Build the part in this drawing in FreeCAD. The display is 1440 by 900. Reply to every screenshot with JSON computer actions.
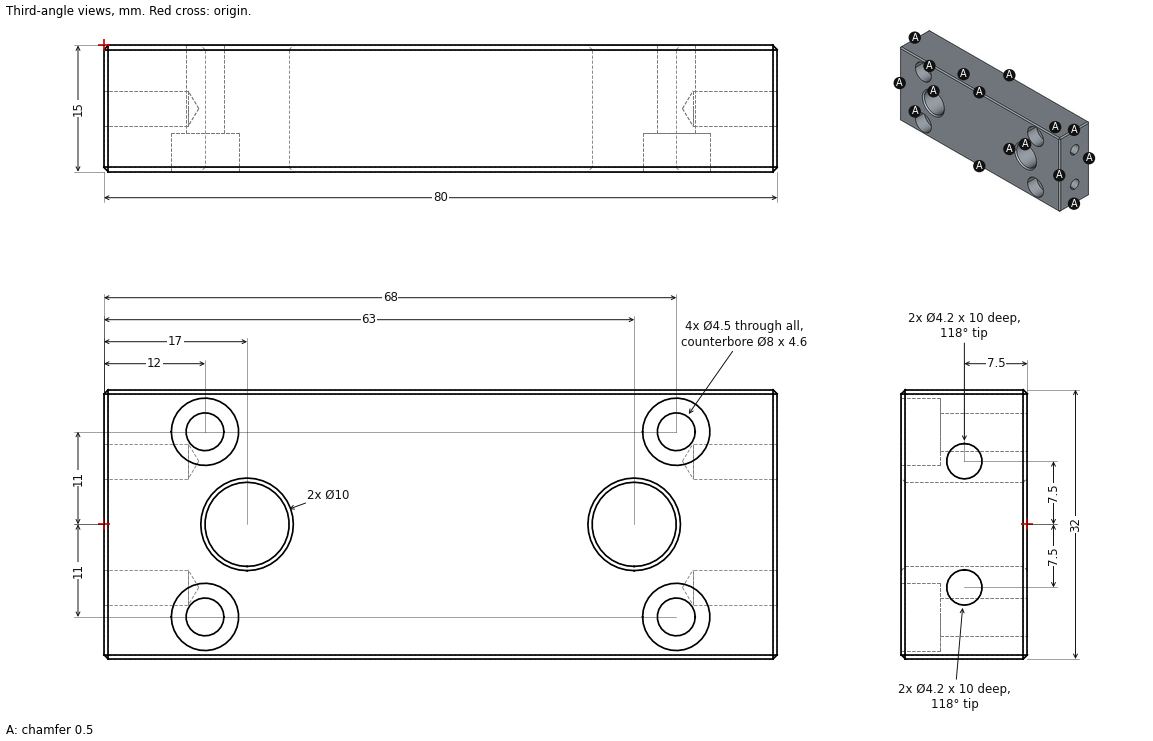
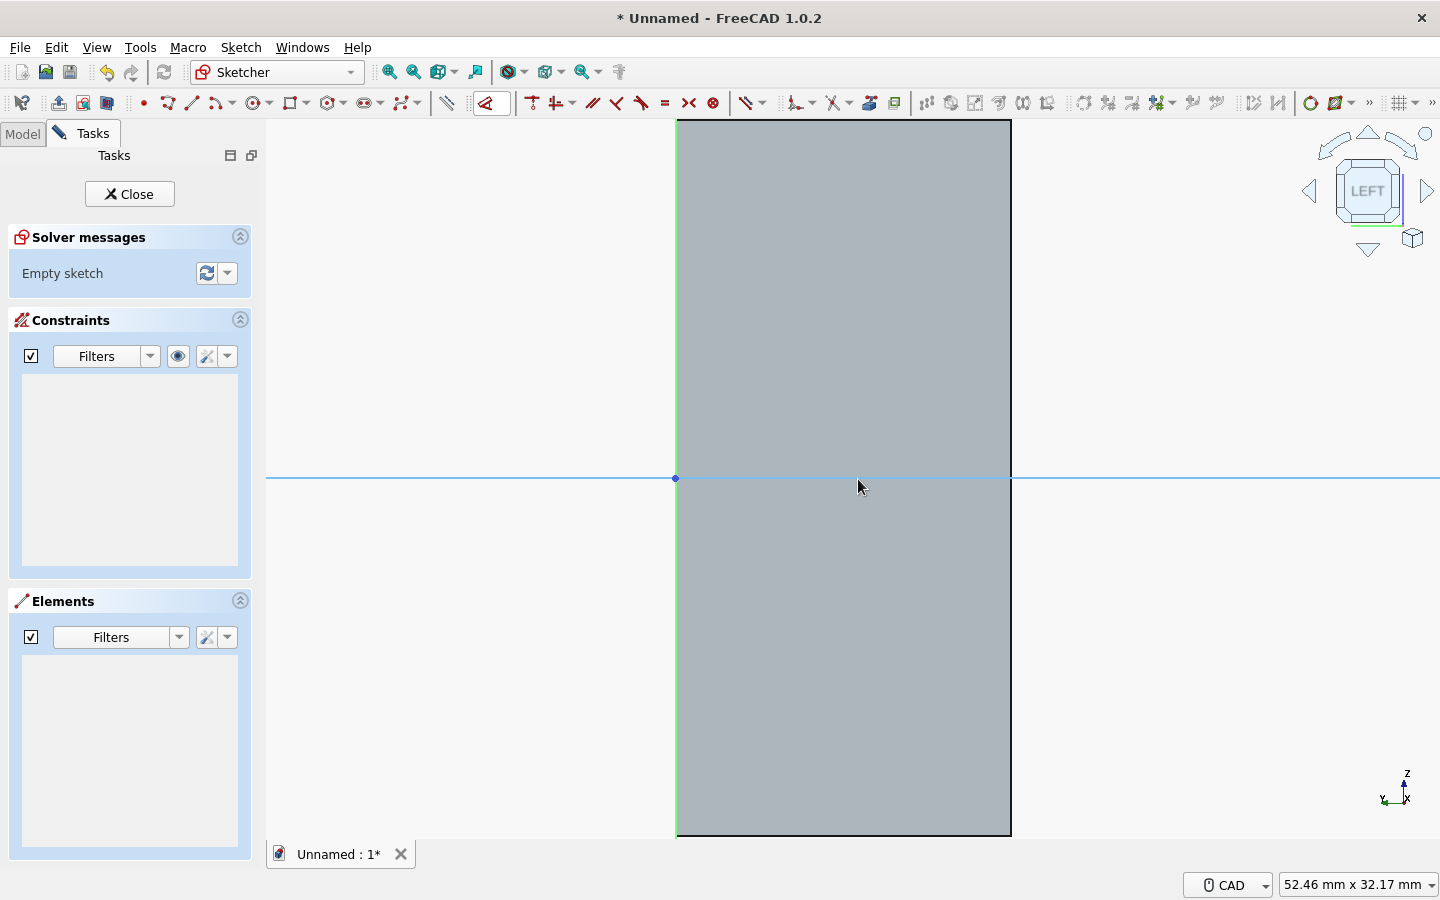
{"action": "left_click", "coordinate": [254, 104]}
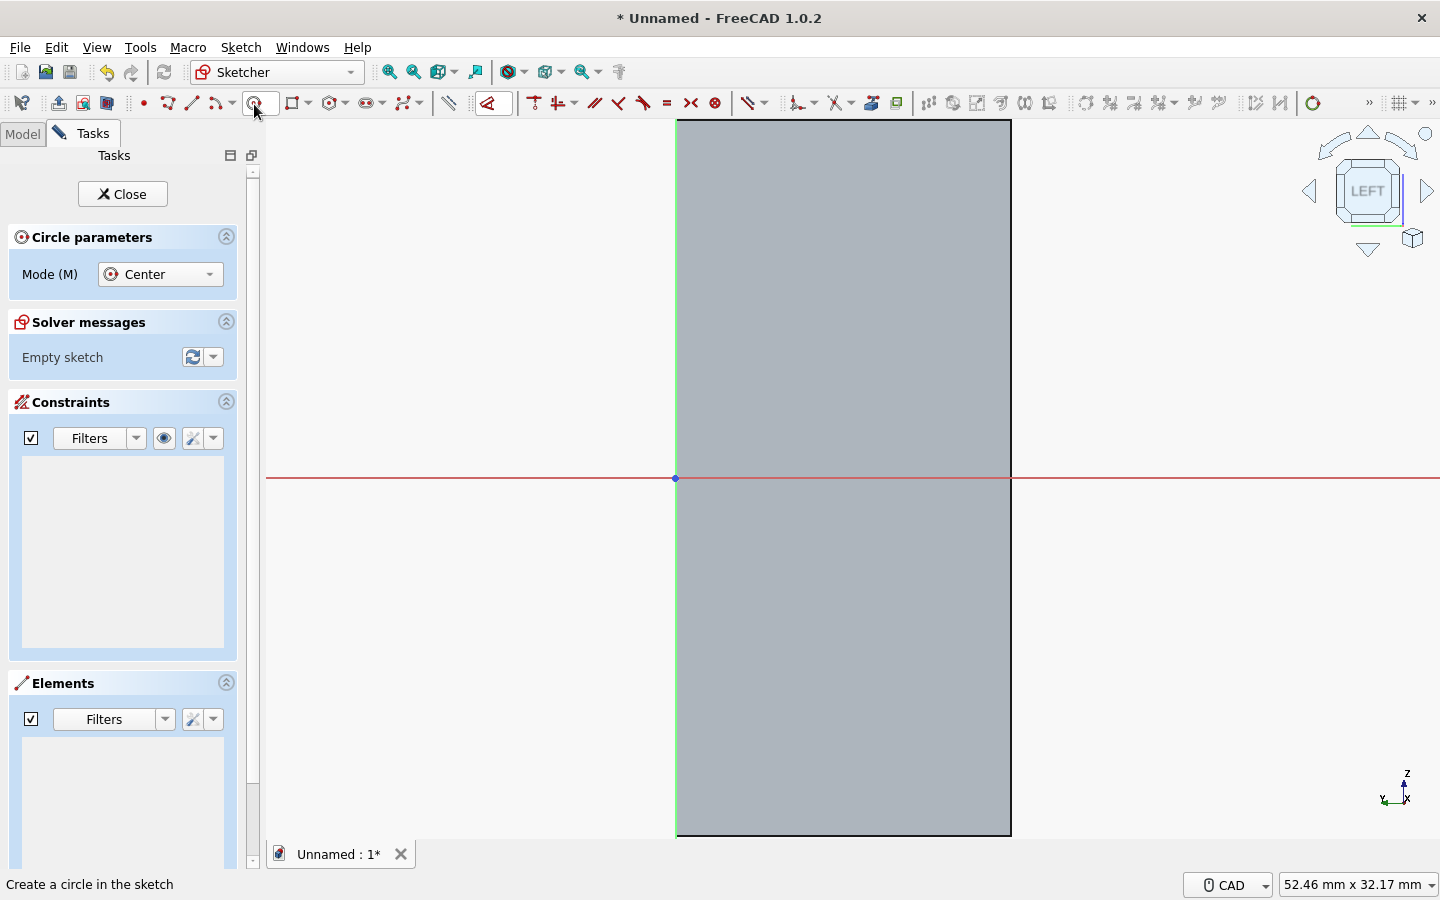
{"action": "left_click", "coordinate": [844, 646]}
{"action": "left_click", "coordinate": [877, 613]}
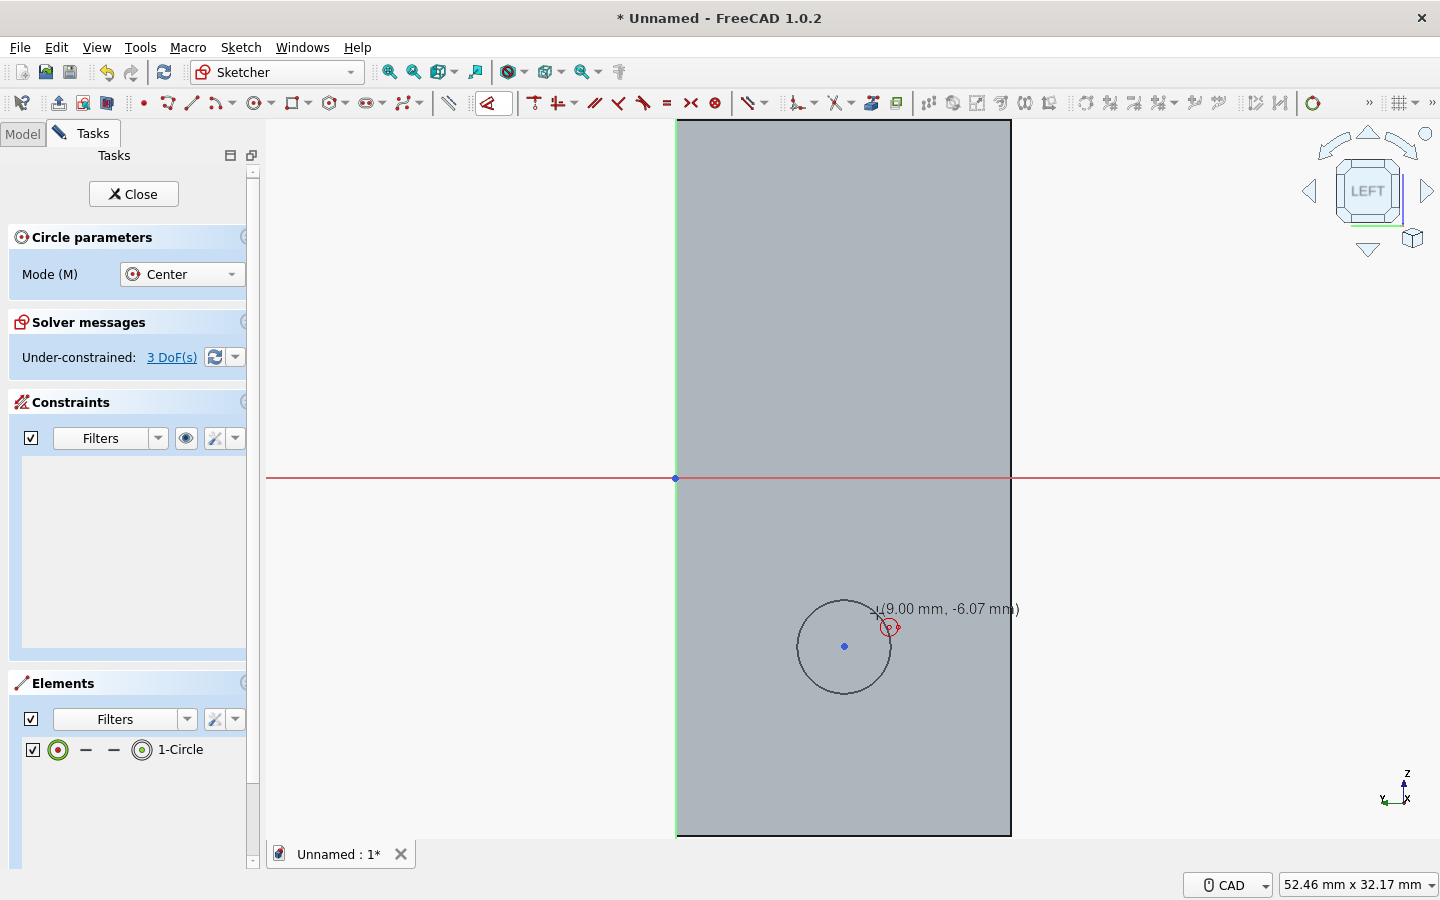
{"action": "left_click", "coordinate": [844, 310]}
{"action": "left_click", "coordinate": [877, 277]}
{"action": "key", "text": "Escape"}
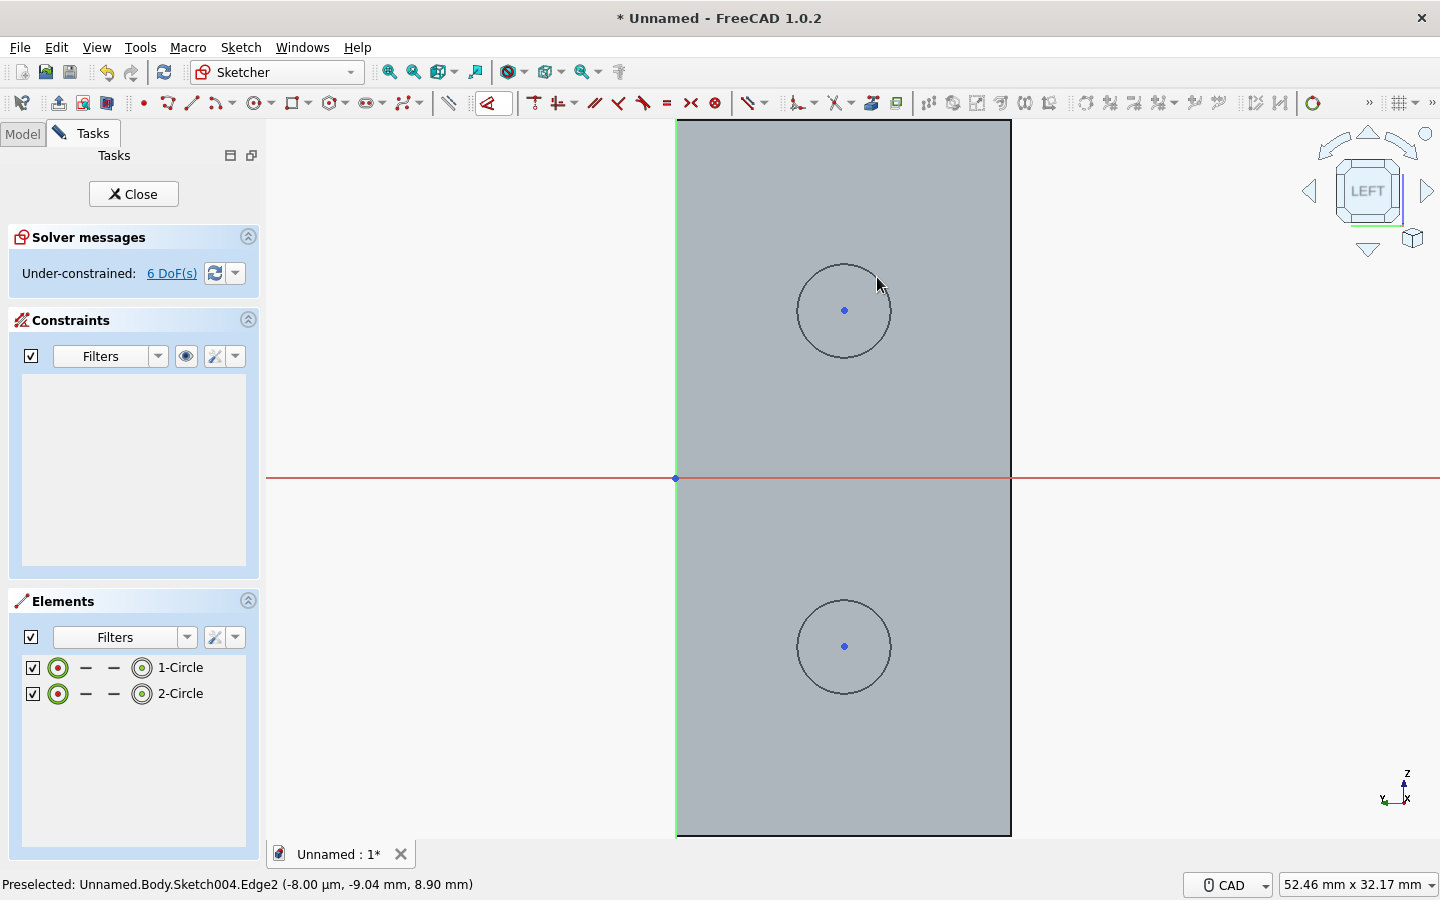
{"action": "left_click", "coordinate": [877, 614]}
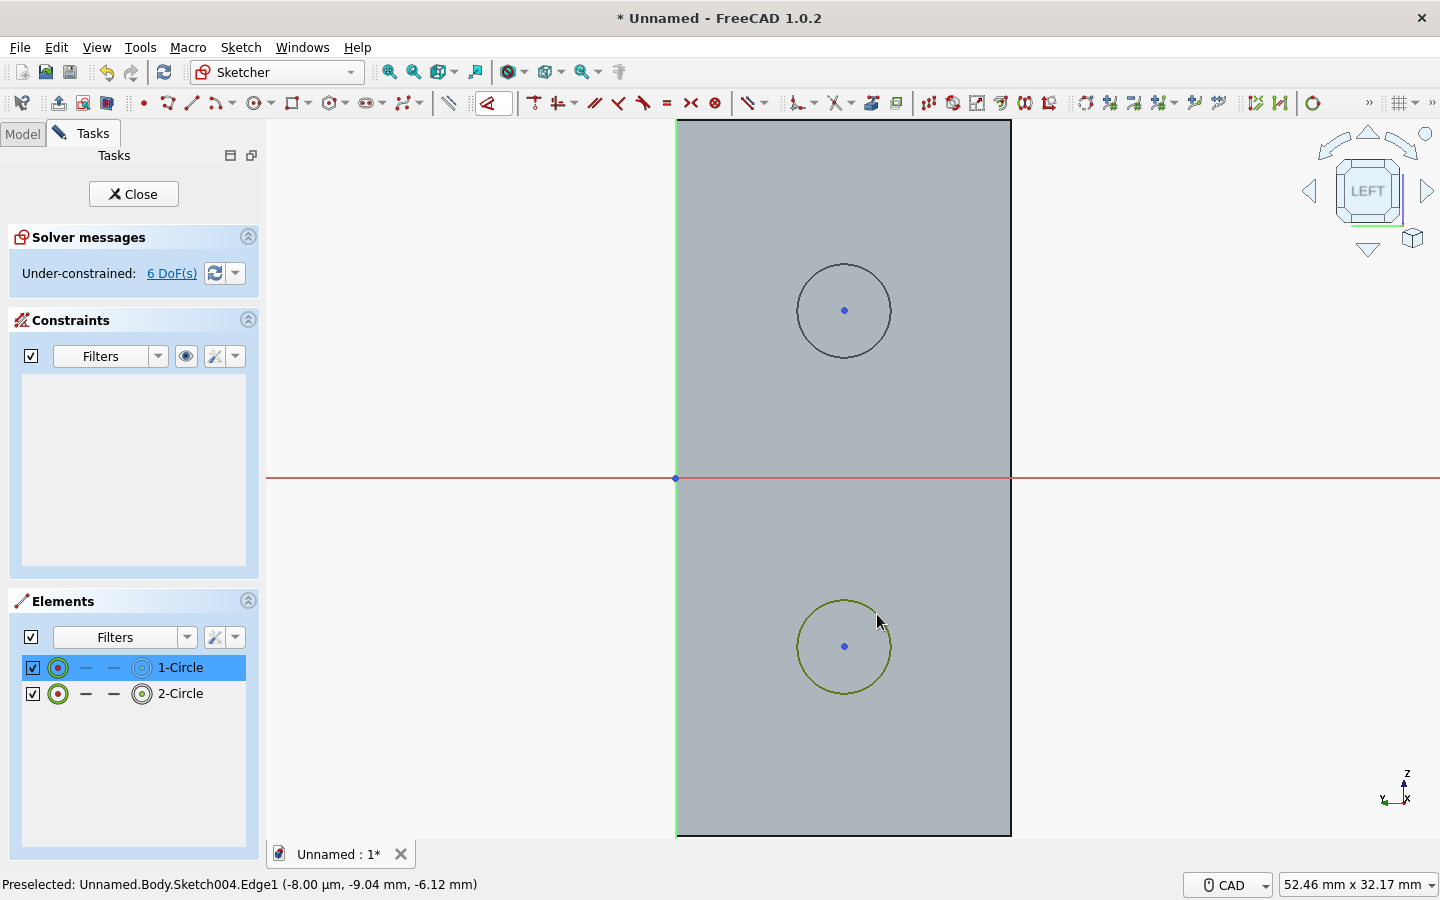
{"action": "left_click", "coordinate": [877, 278]}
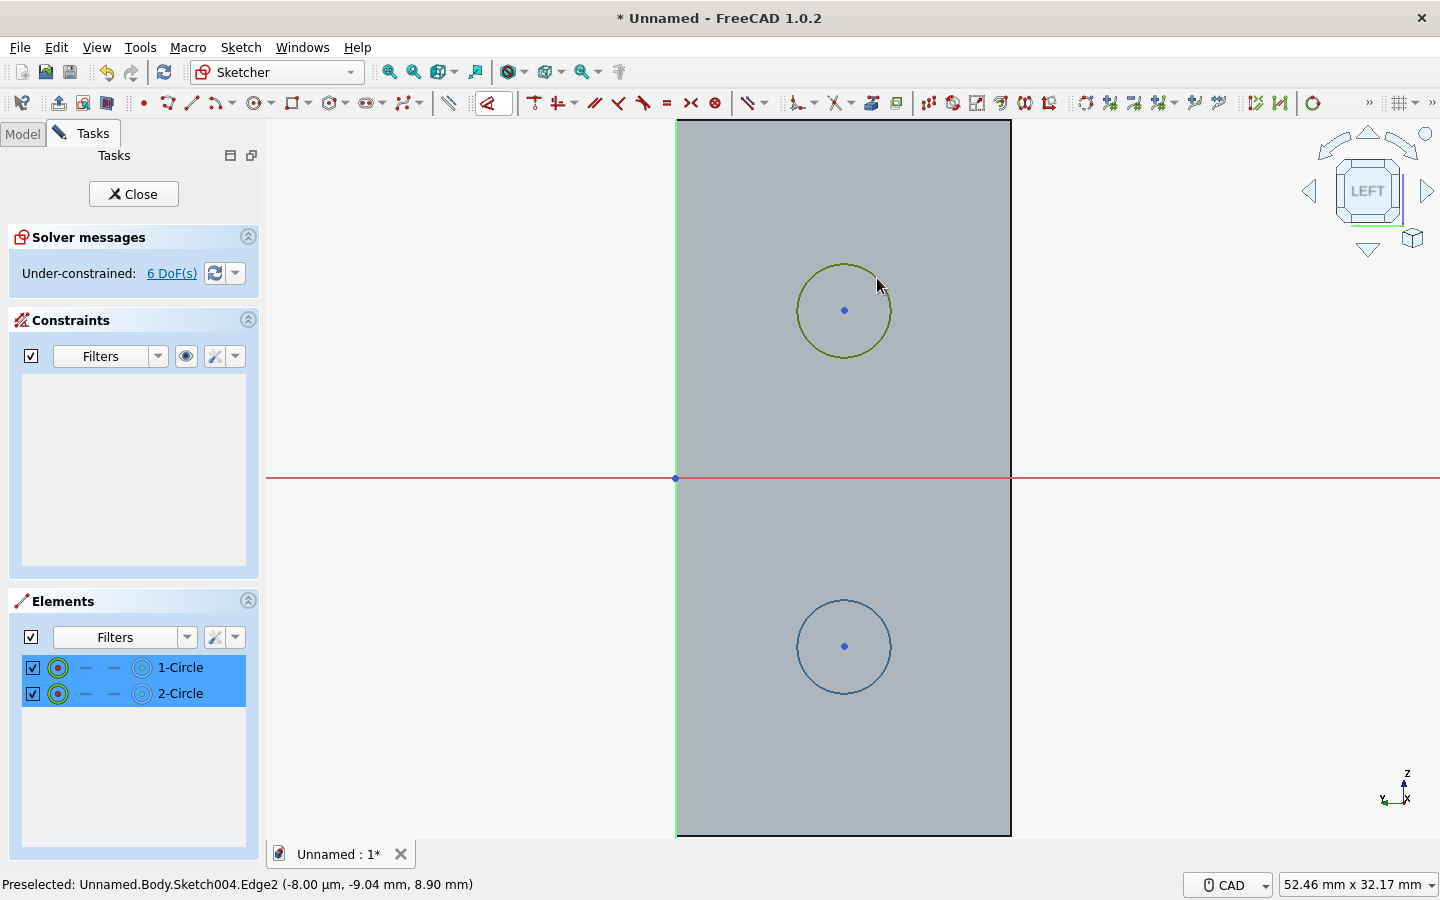
{"action": "left_click", "coordinate": [668, 104]}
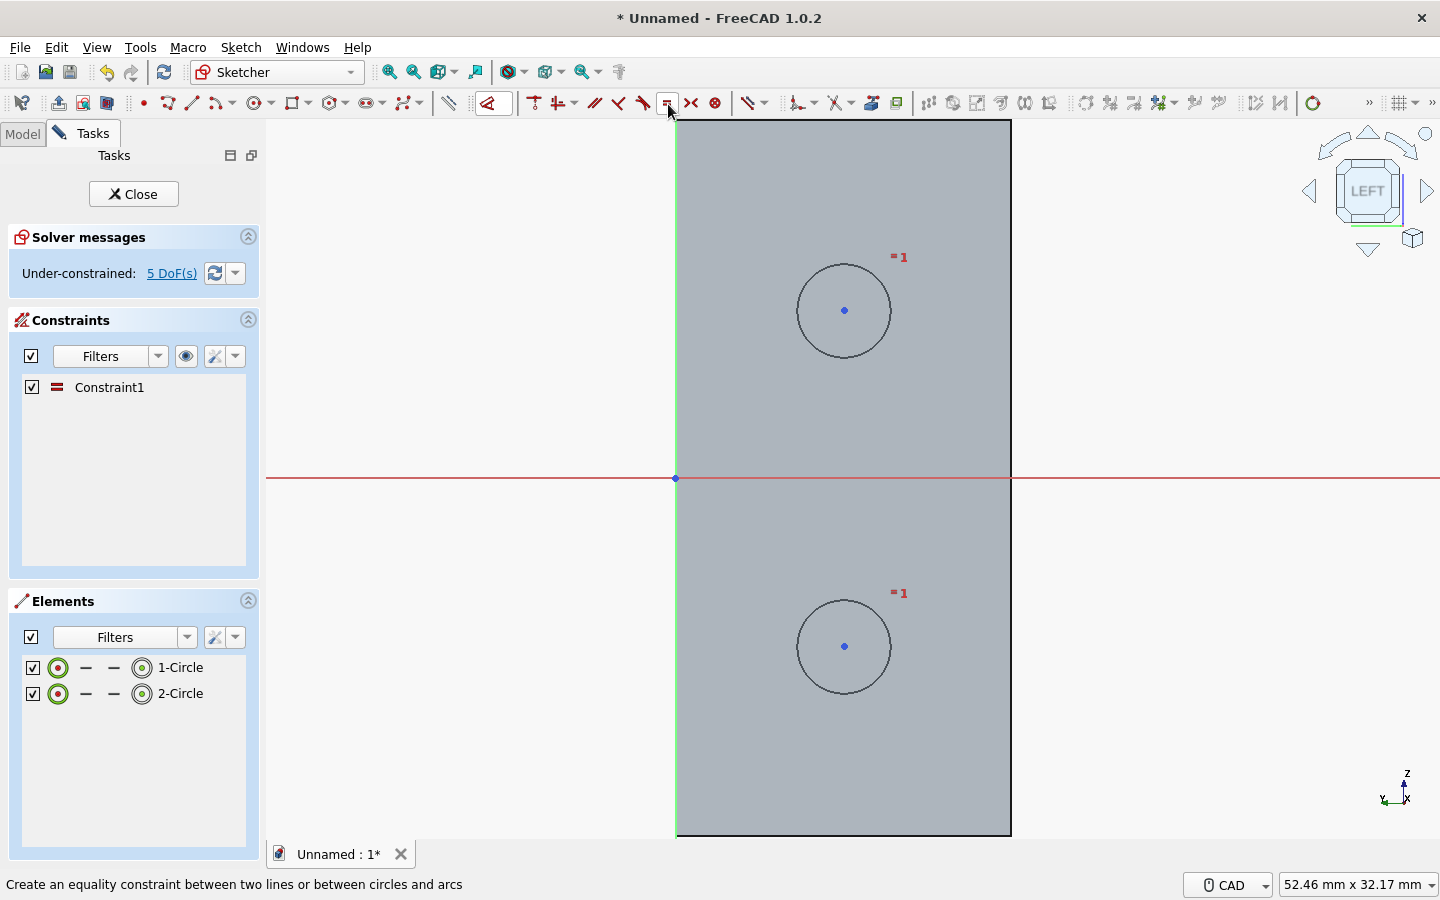
{"action": "left_click", "coordinate": [877, 614]}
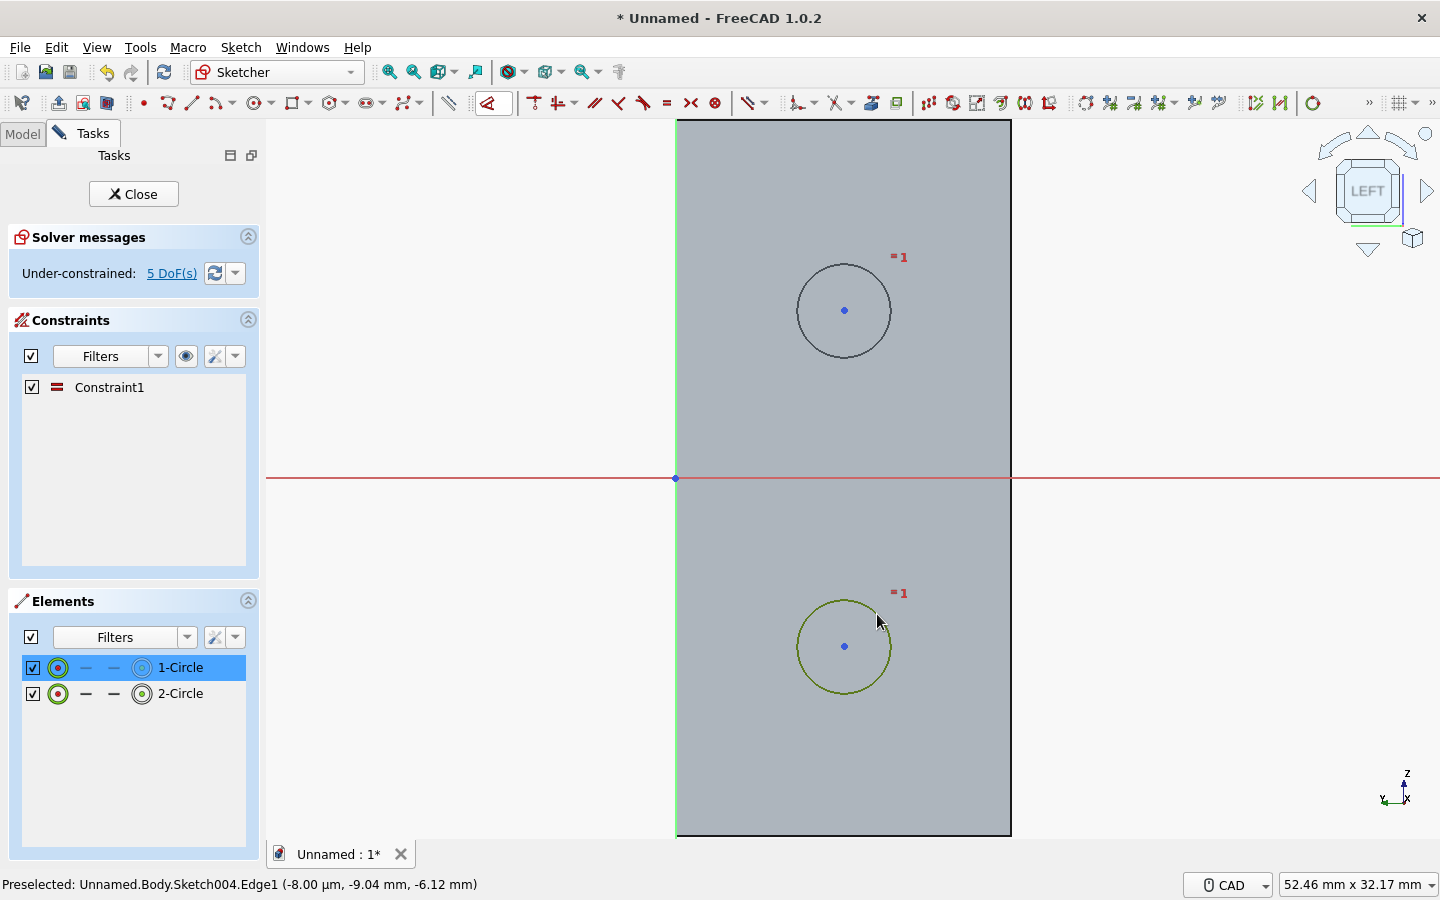
{"action": "left_click", "coordinate": [506, 104]}